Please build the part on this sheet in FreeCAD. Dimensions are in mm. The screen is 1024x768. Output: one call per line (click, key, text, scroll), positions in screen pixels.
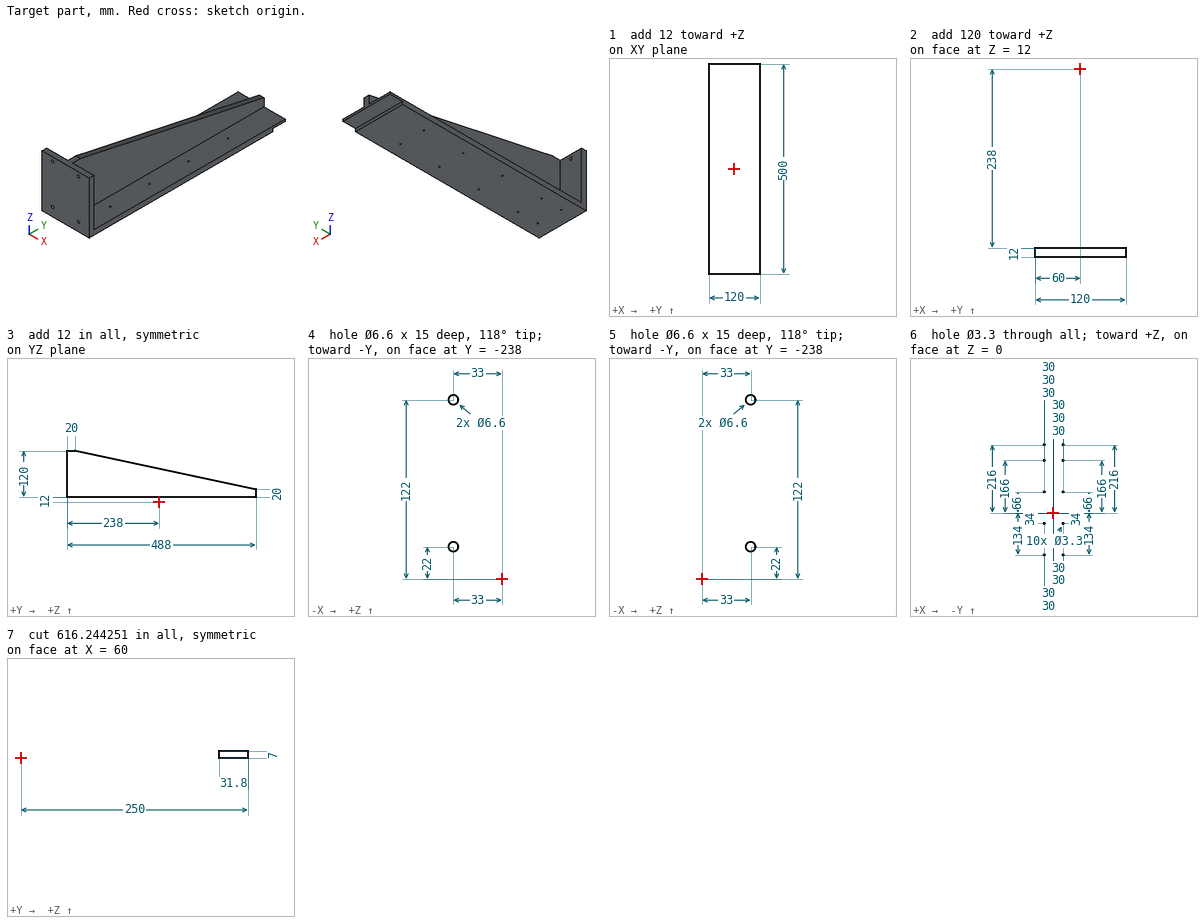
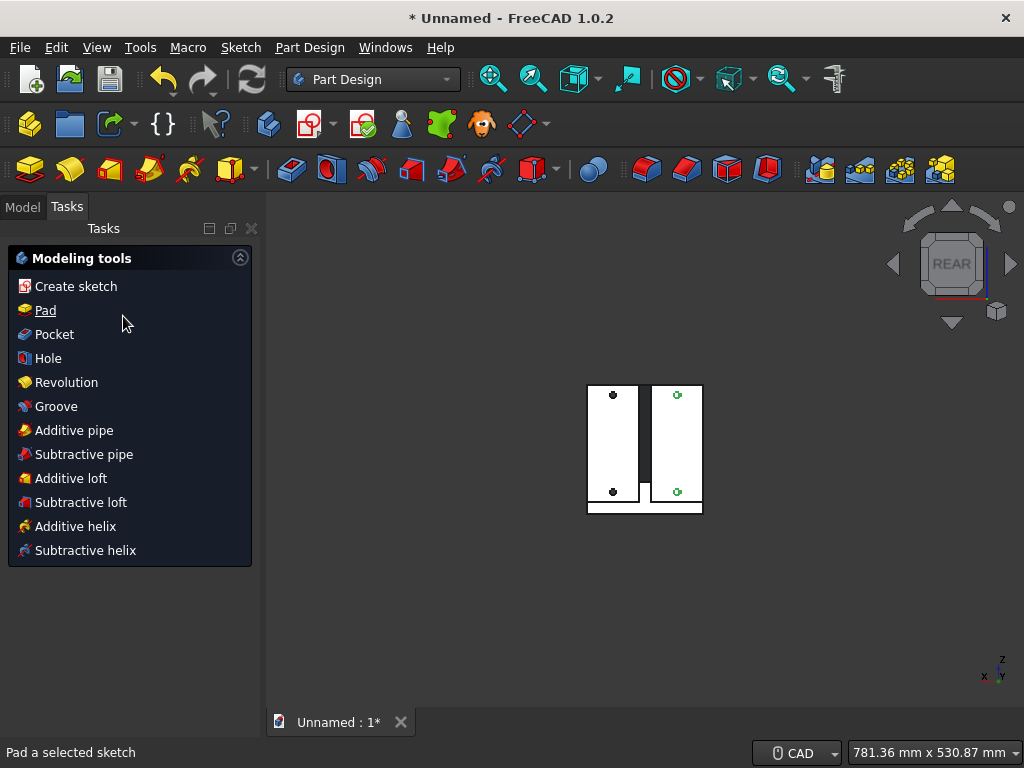
click(332, 170)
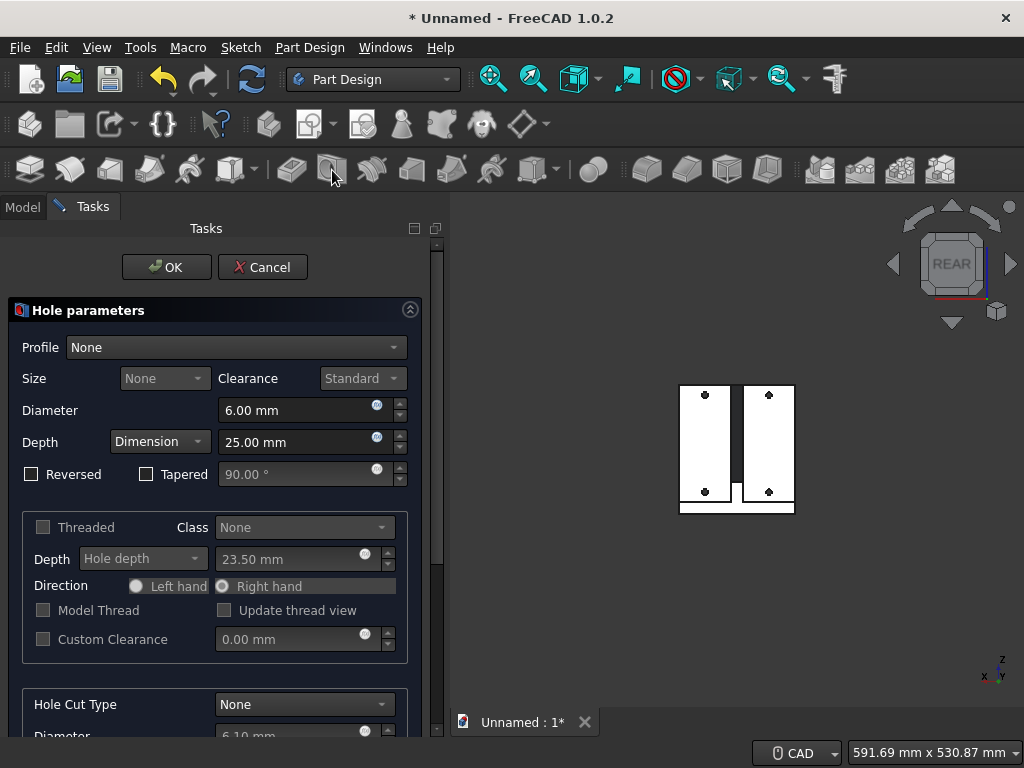
triple_click(305, 410)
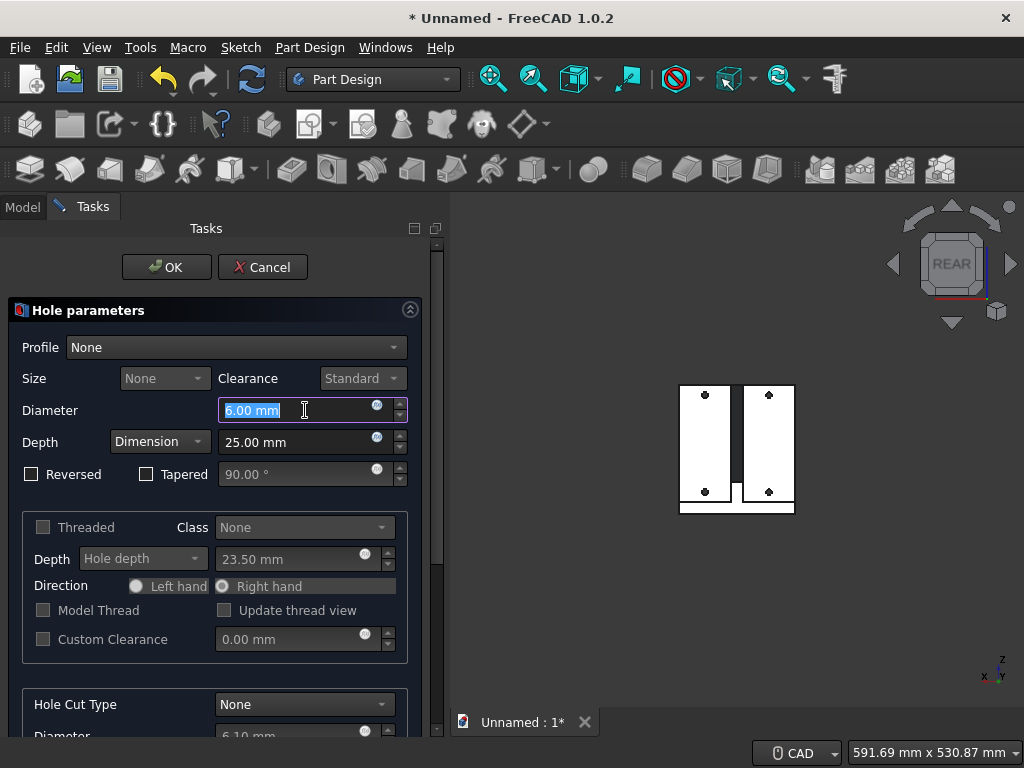
text(6.6)
key(Tab)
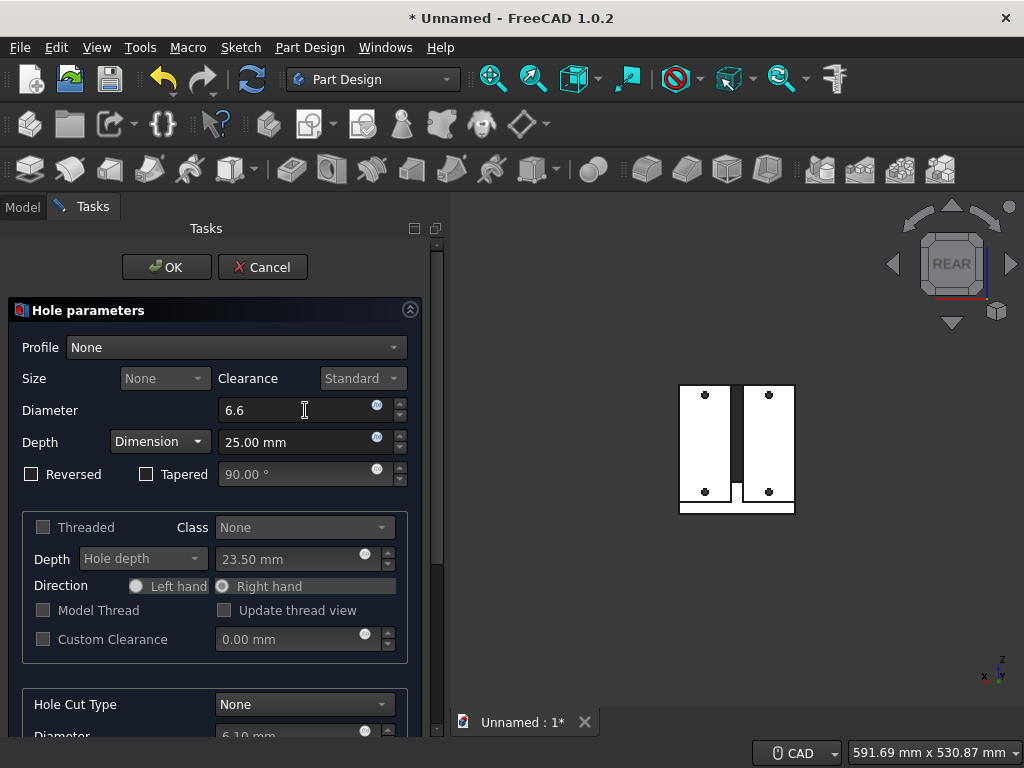
triple_click(305, 442)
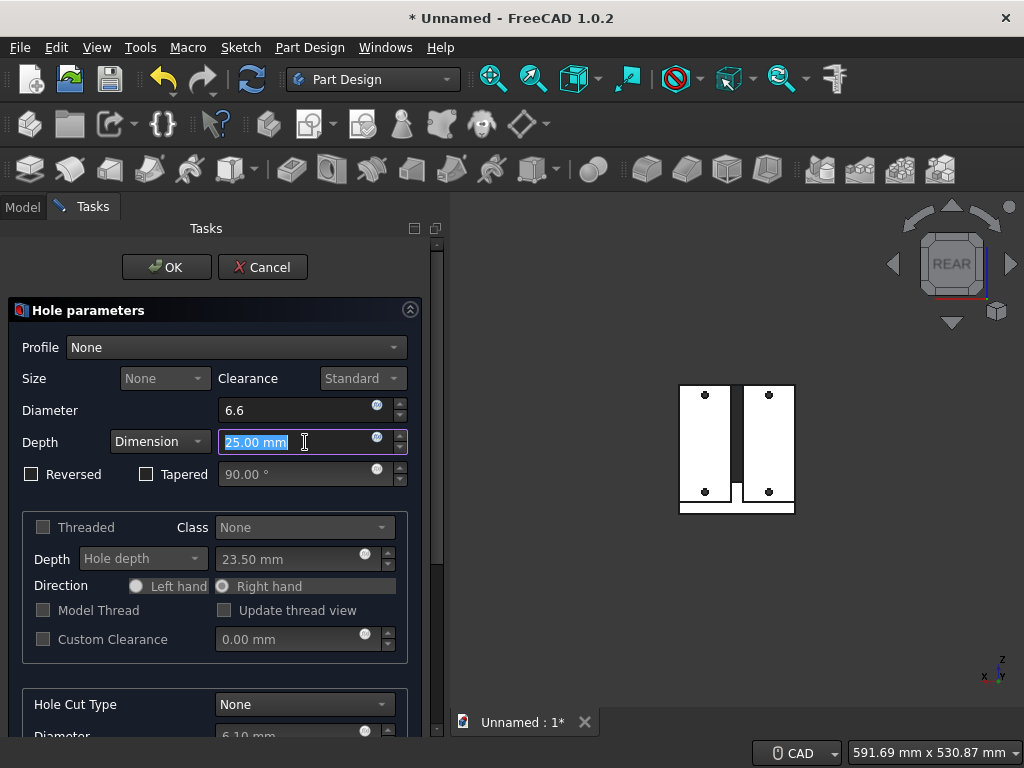
text(15)
key(Tab)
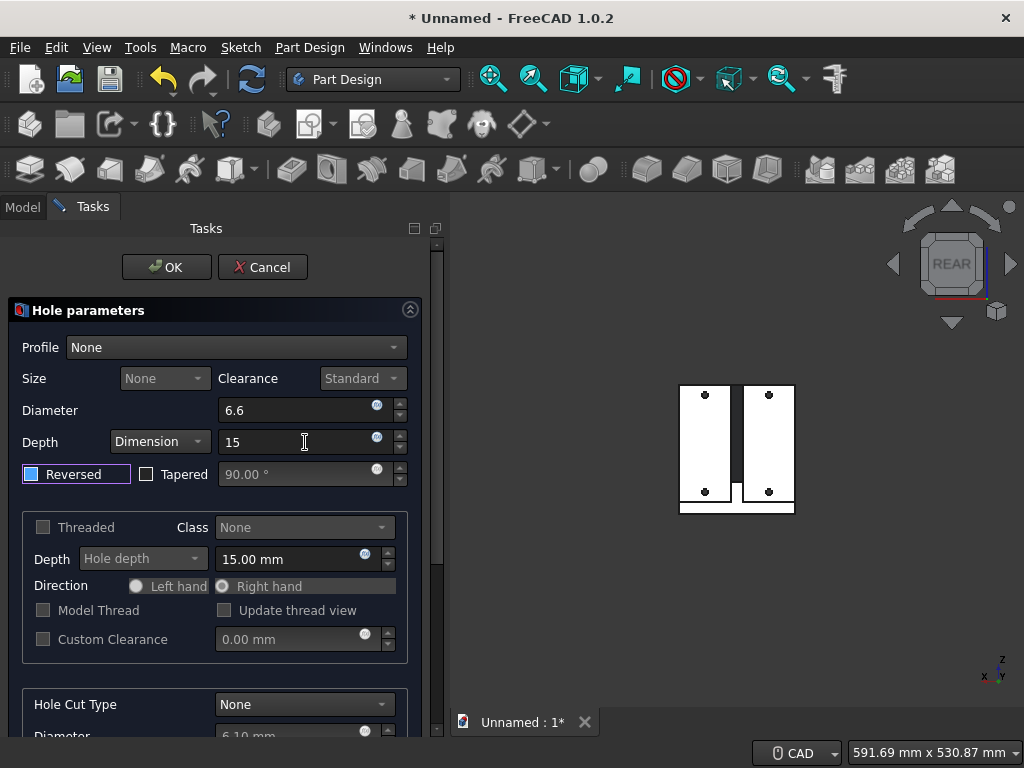
click(167, 267)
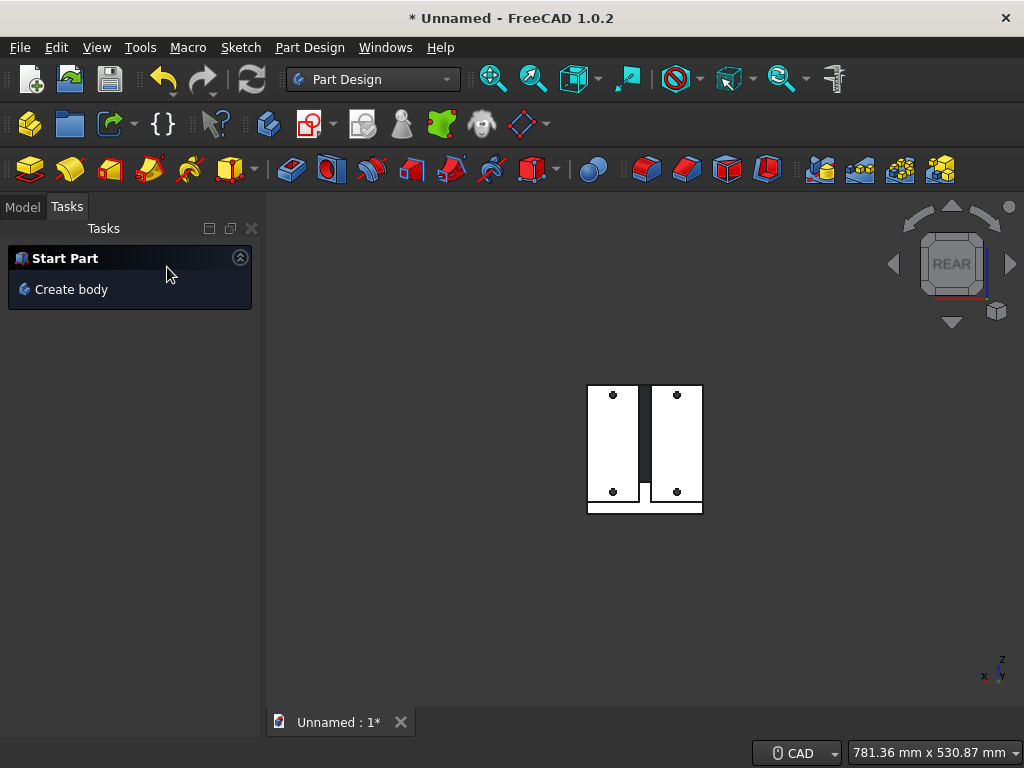
click(494, 80)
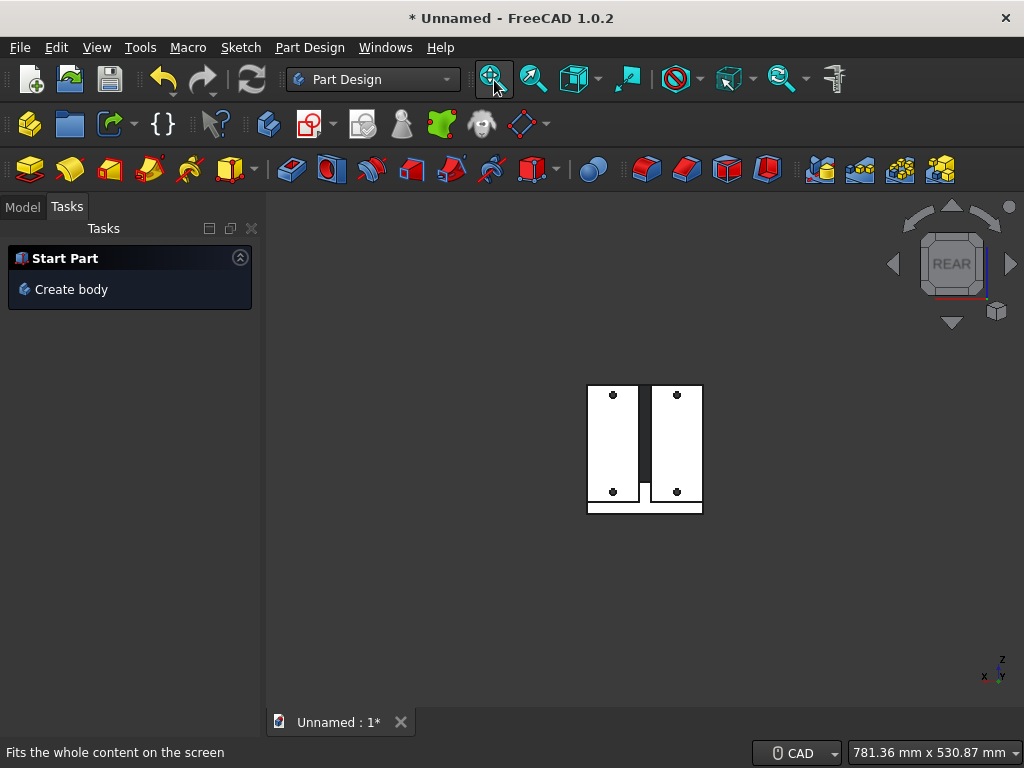
key(5)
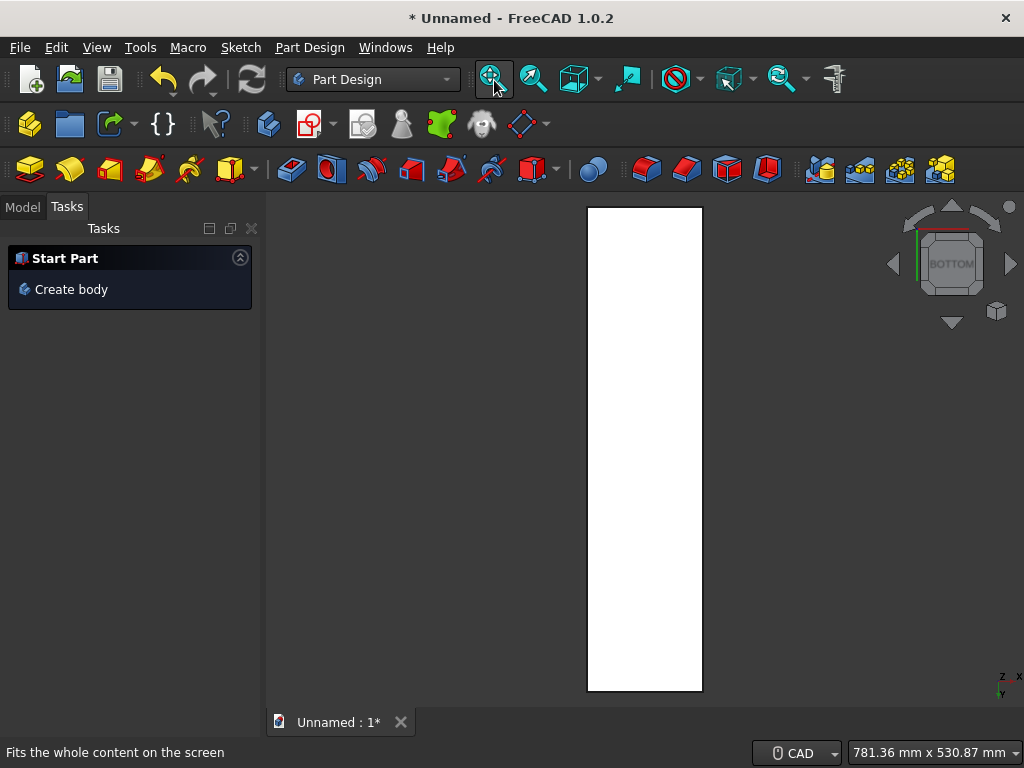
click(645, 587)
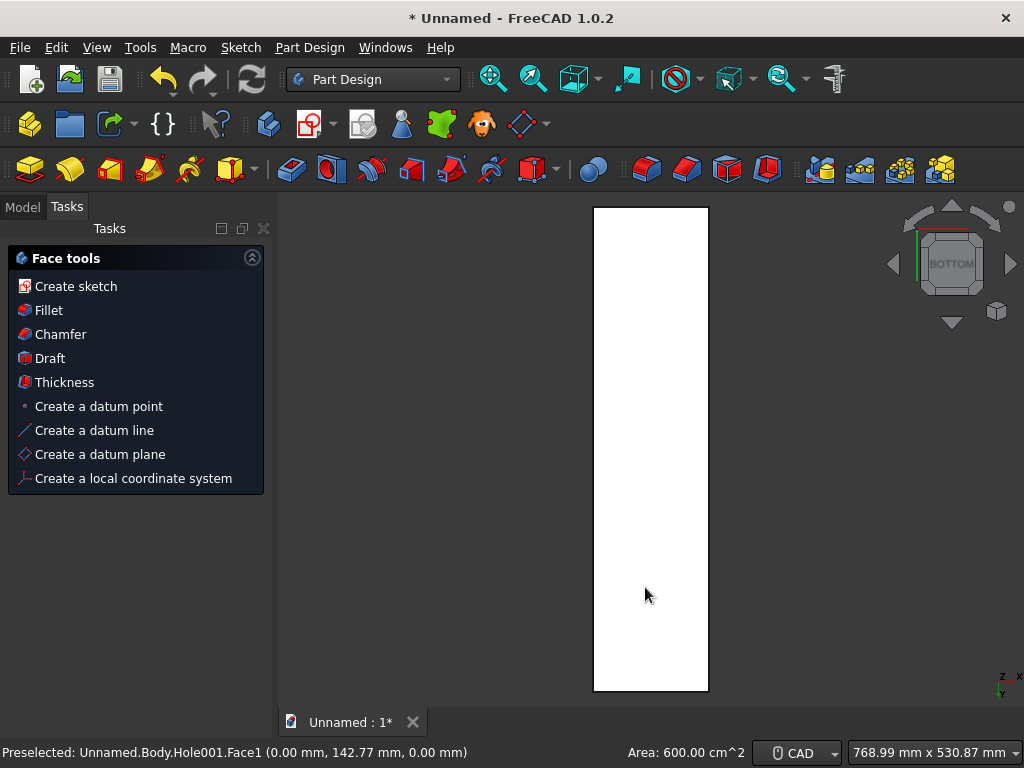
click(310, 124)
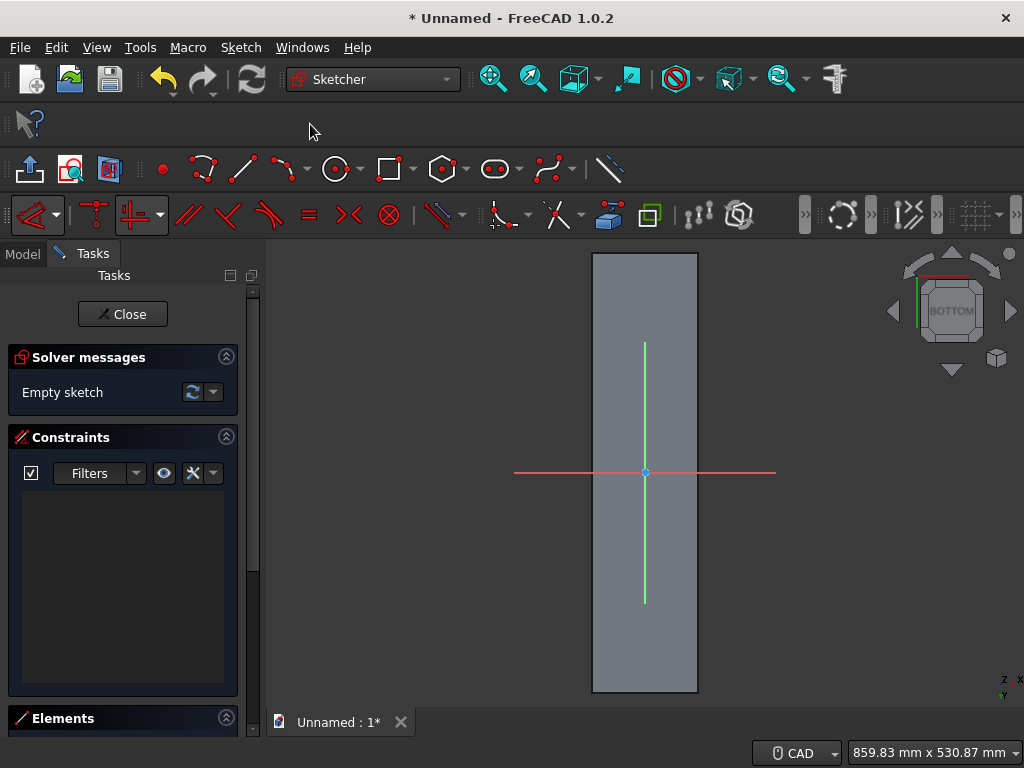
scroll(294, 636, down, 1)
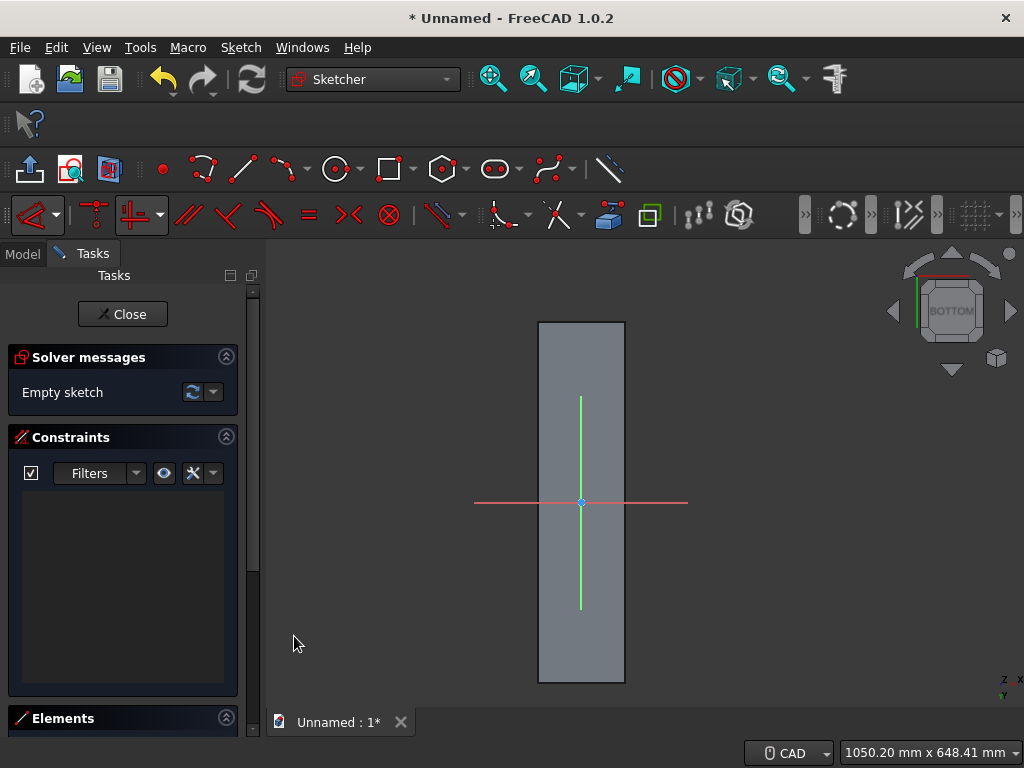
click(336, 170)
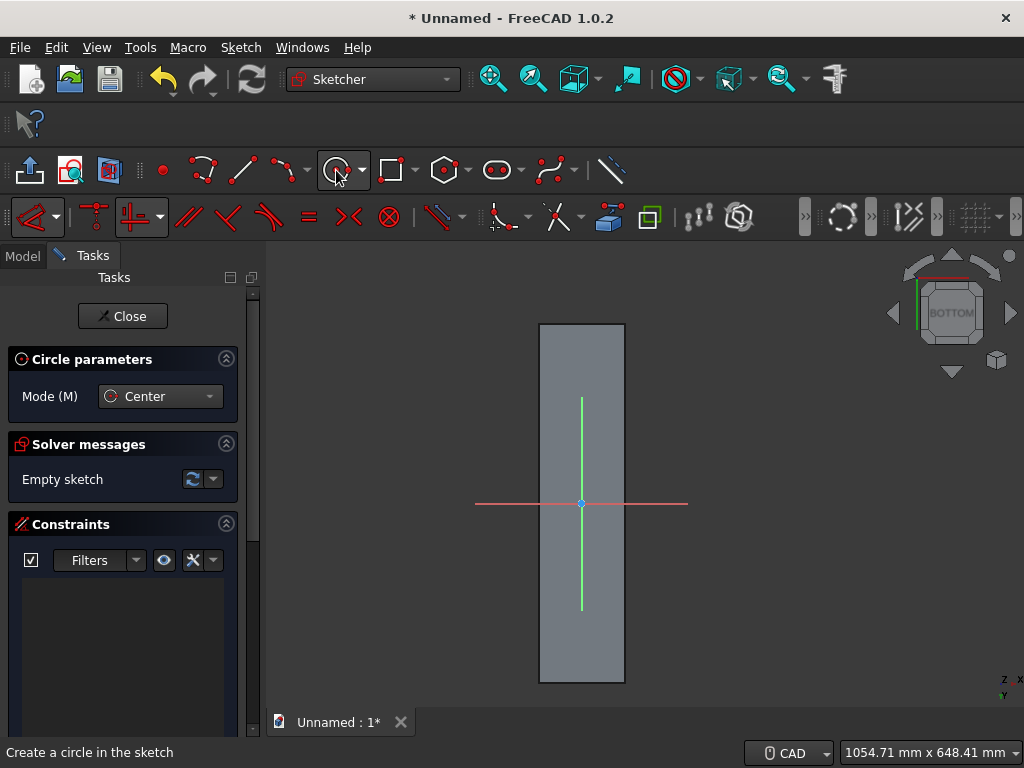
scroll(603, 528, up, 15)